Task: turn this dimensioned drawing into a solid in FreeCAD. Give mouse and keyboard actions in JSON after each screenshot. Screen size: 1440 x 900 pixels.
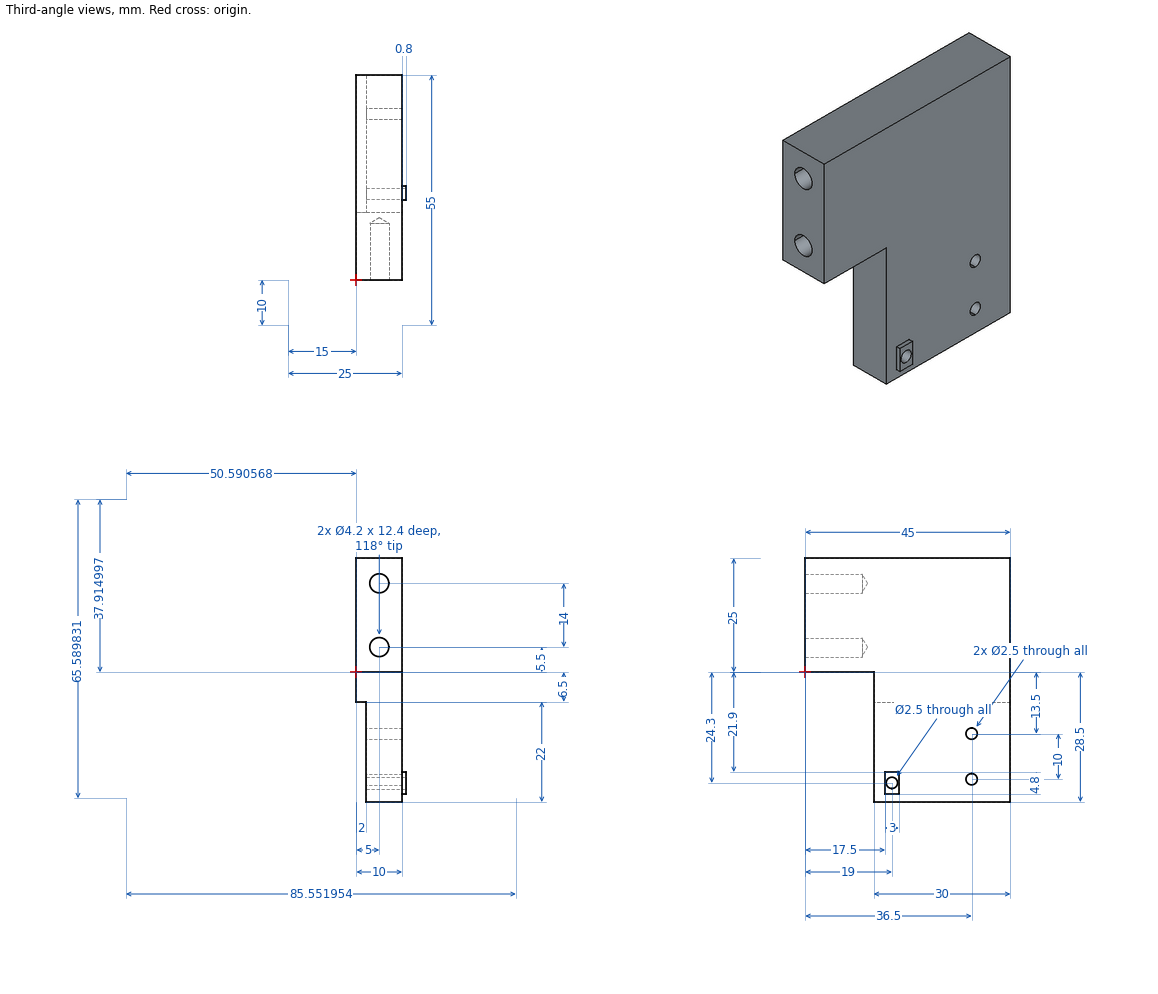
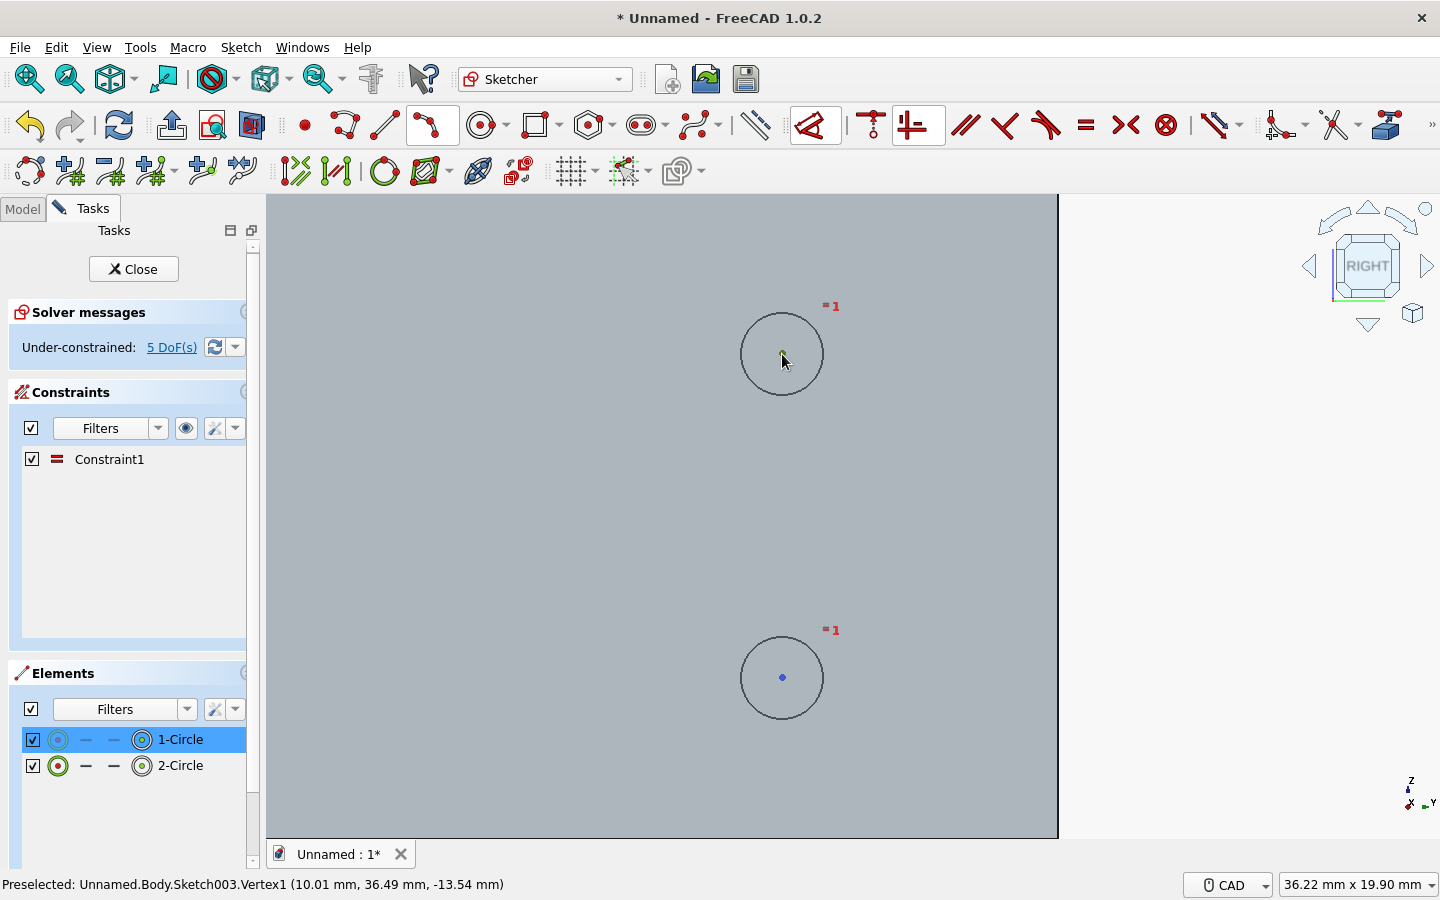
{"action": "left_click", "coordinate": [782, 678]}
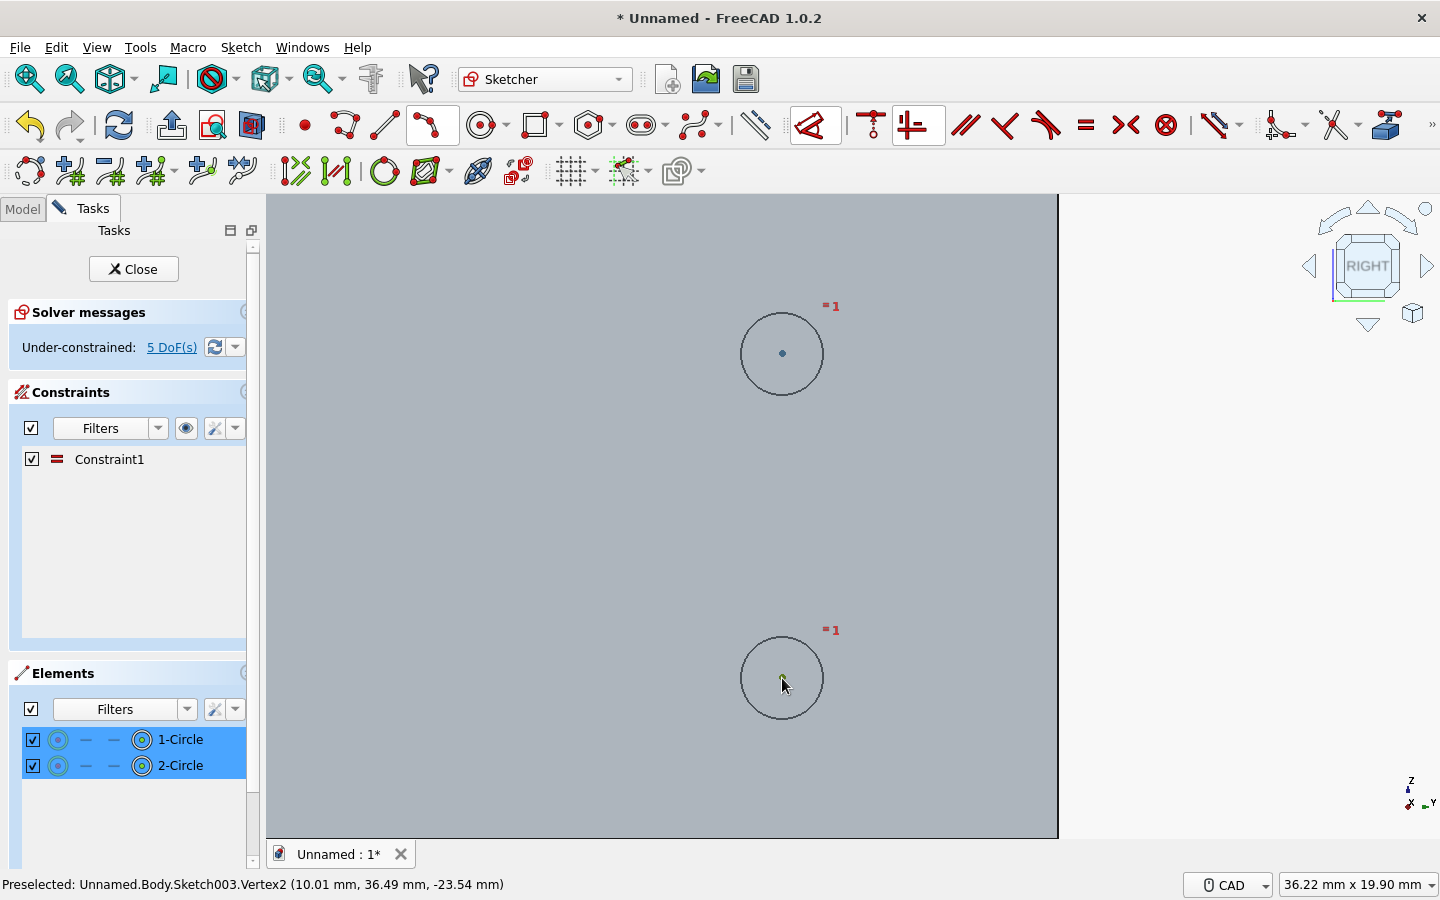
{"action": "key", "text": "v"}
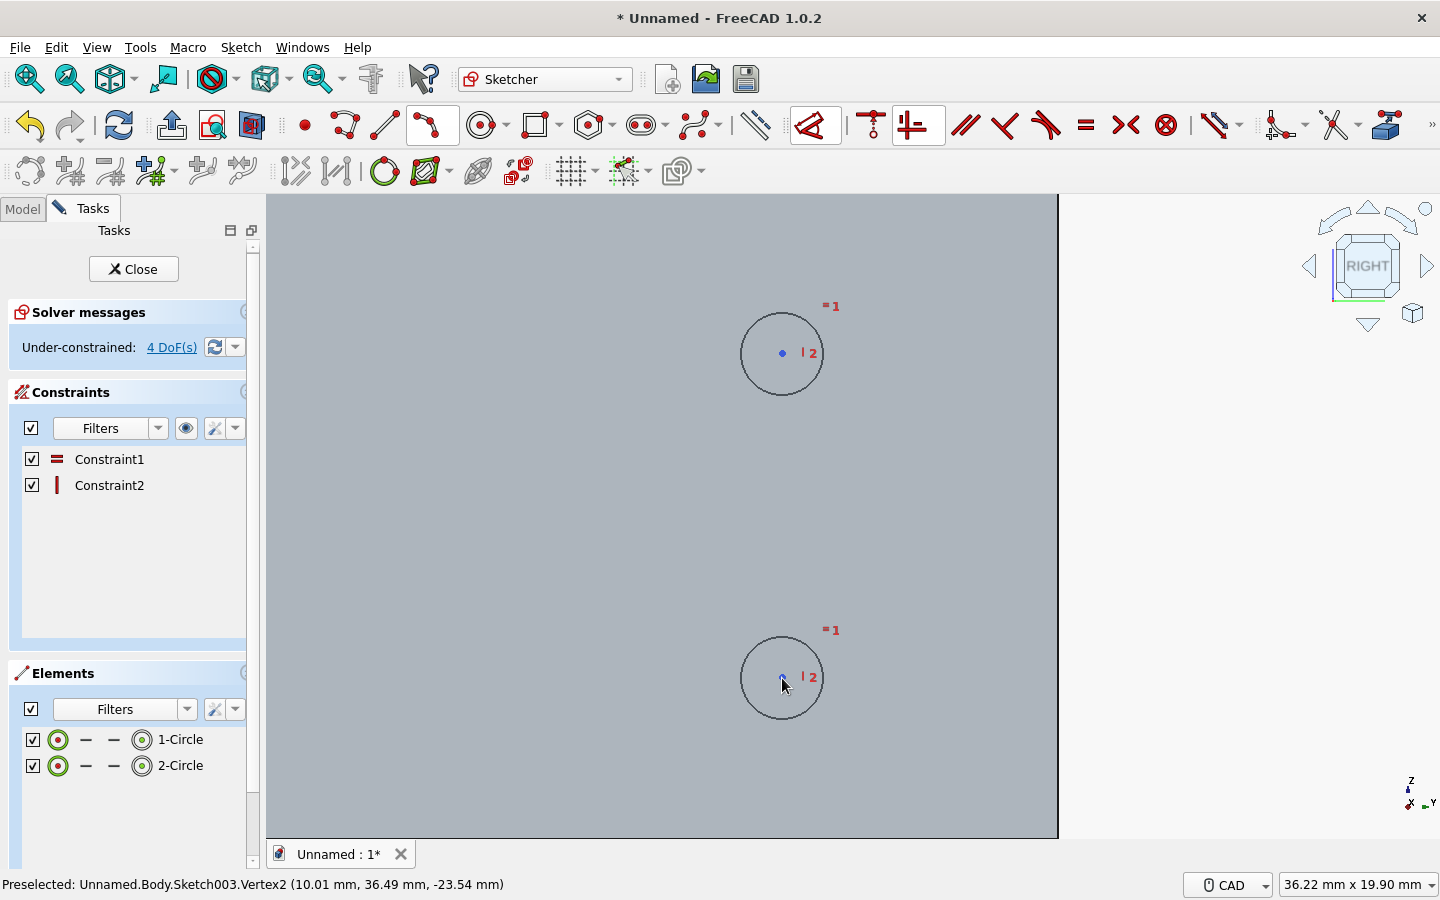
{"action": "left_click", "coordinate": [811, 325]}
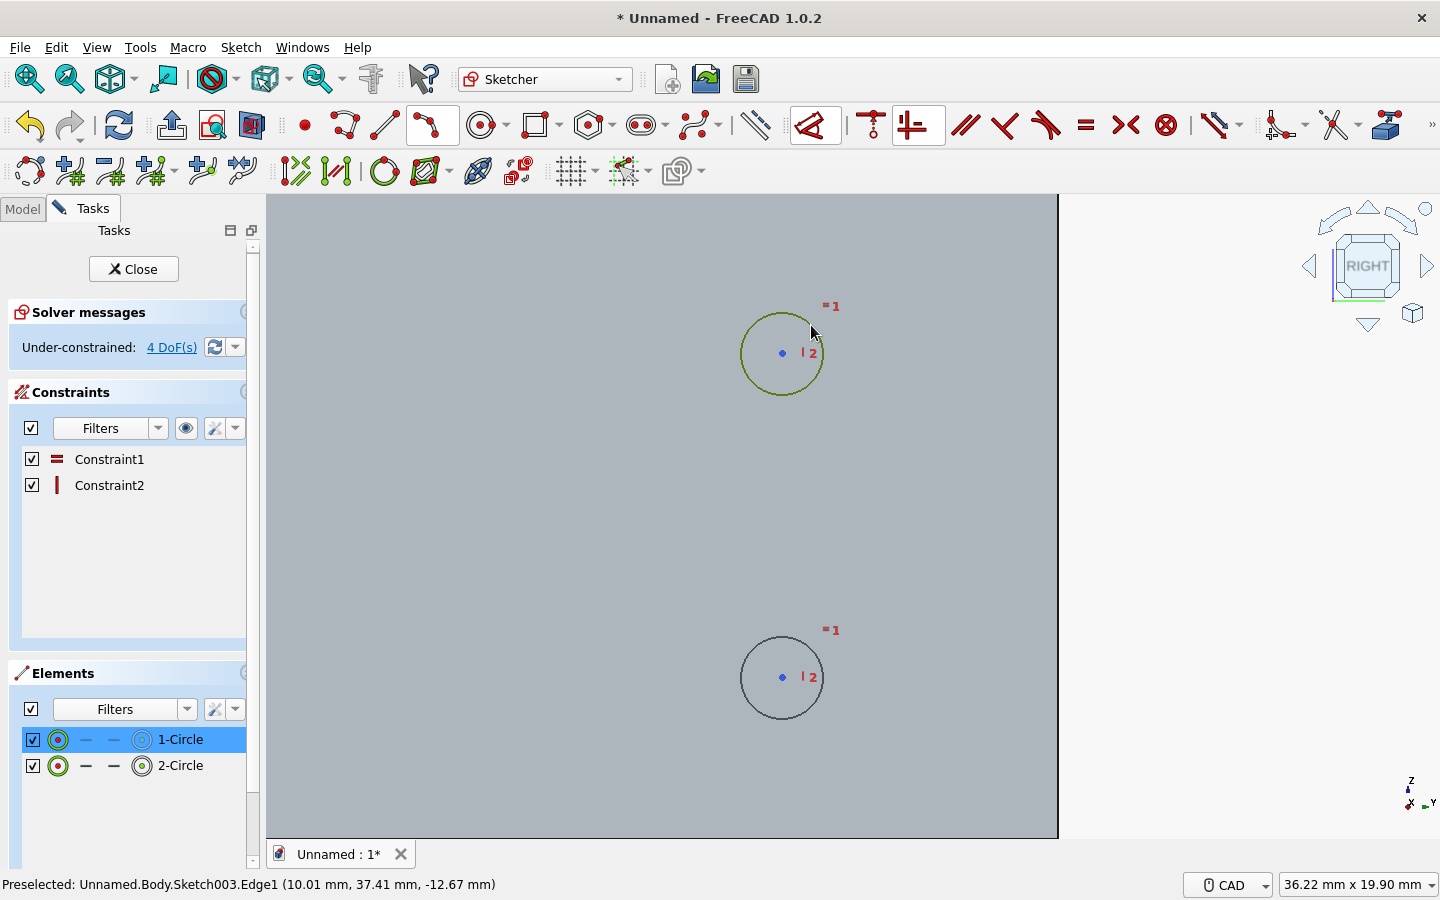
{"action": "left_click", "coordinate": [836, 126]}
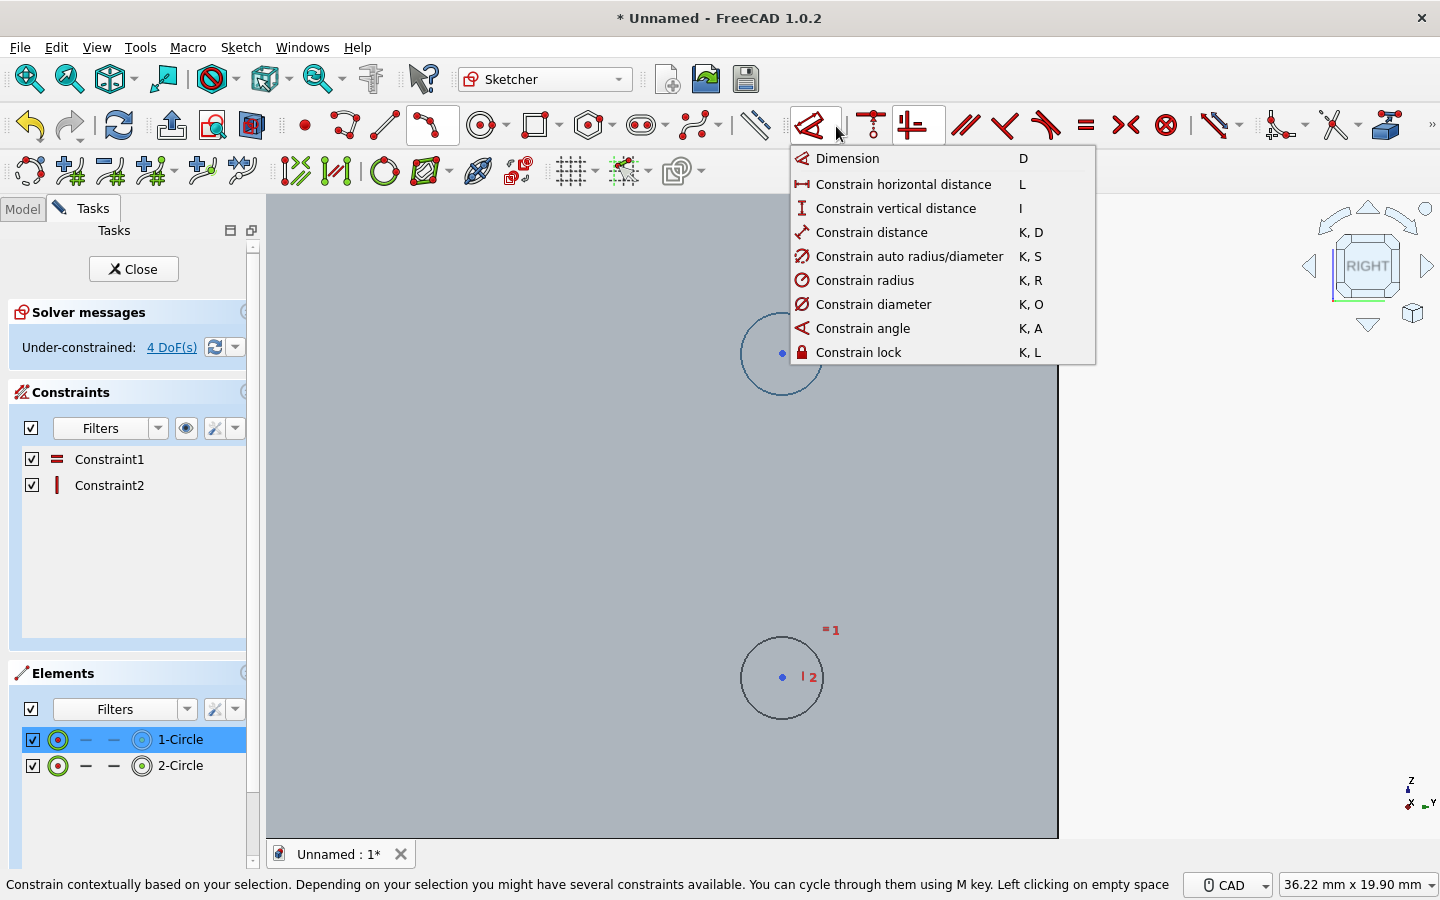
{"action": "left_click", "coordinate": [943, 304]}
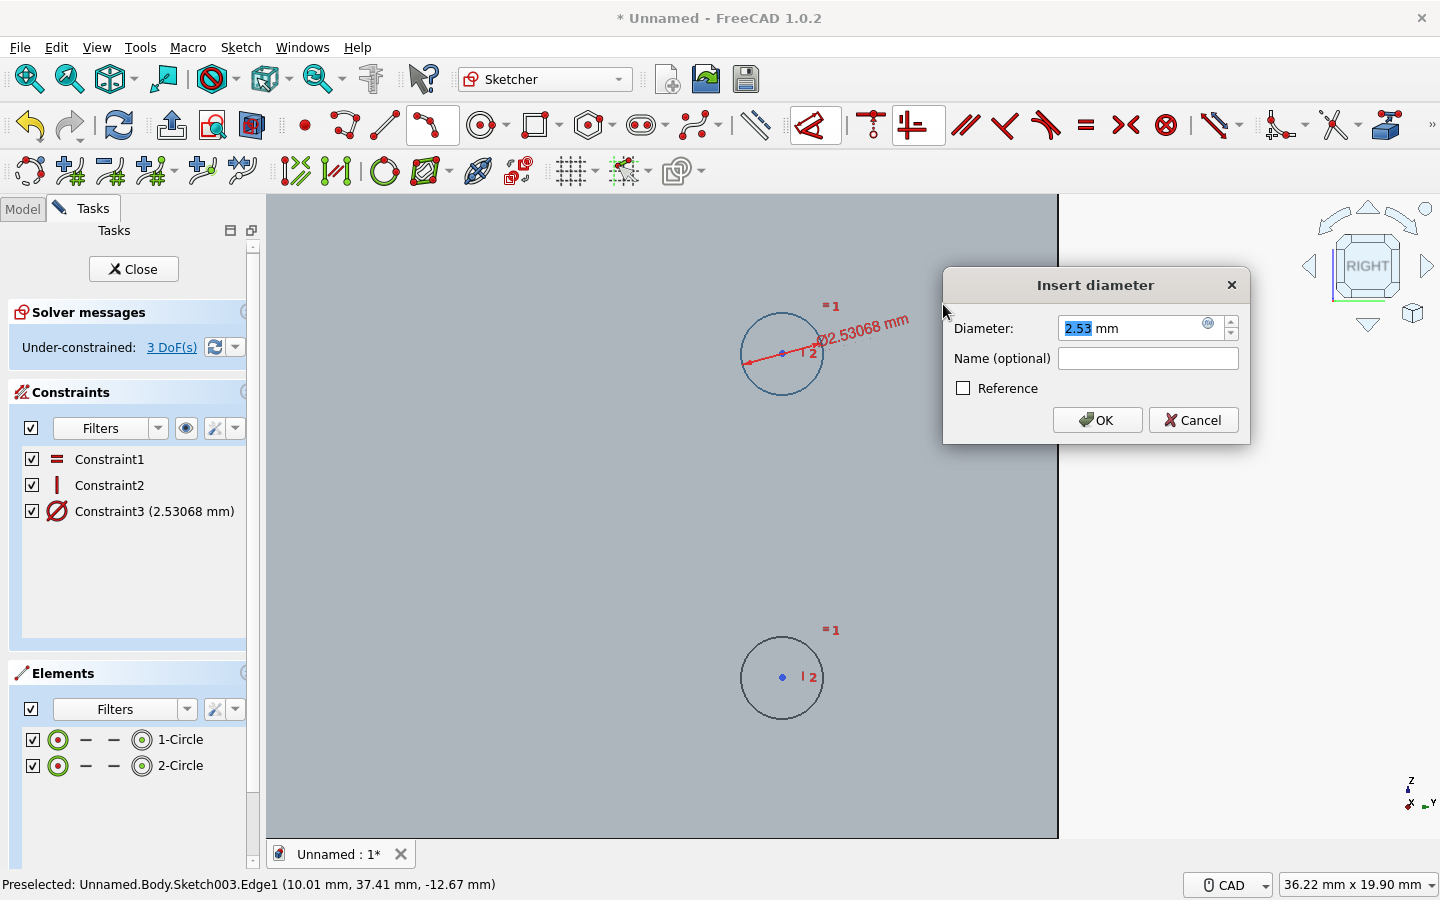
{"action": "type", "text": "2.5"}
{"action": "key", "text": "Return"}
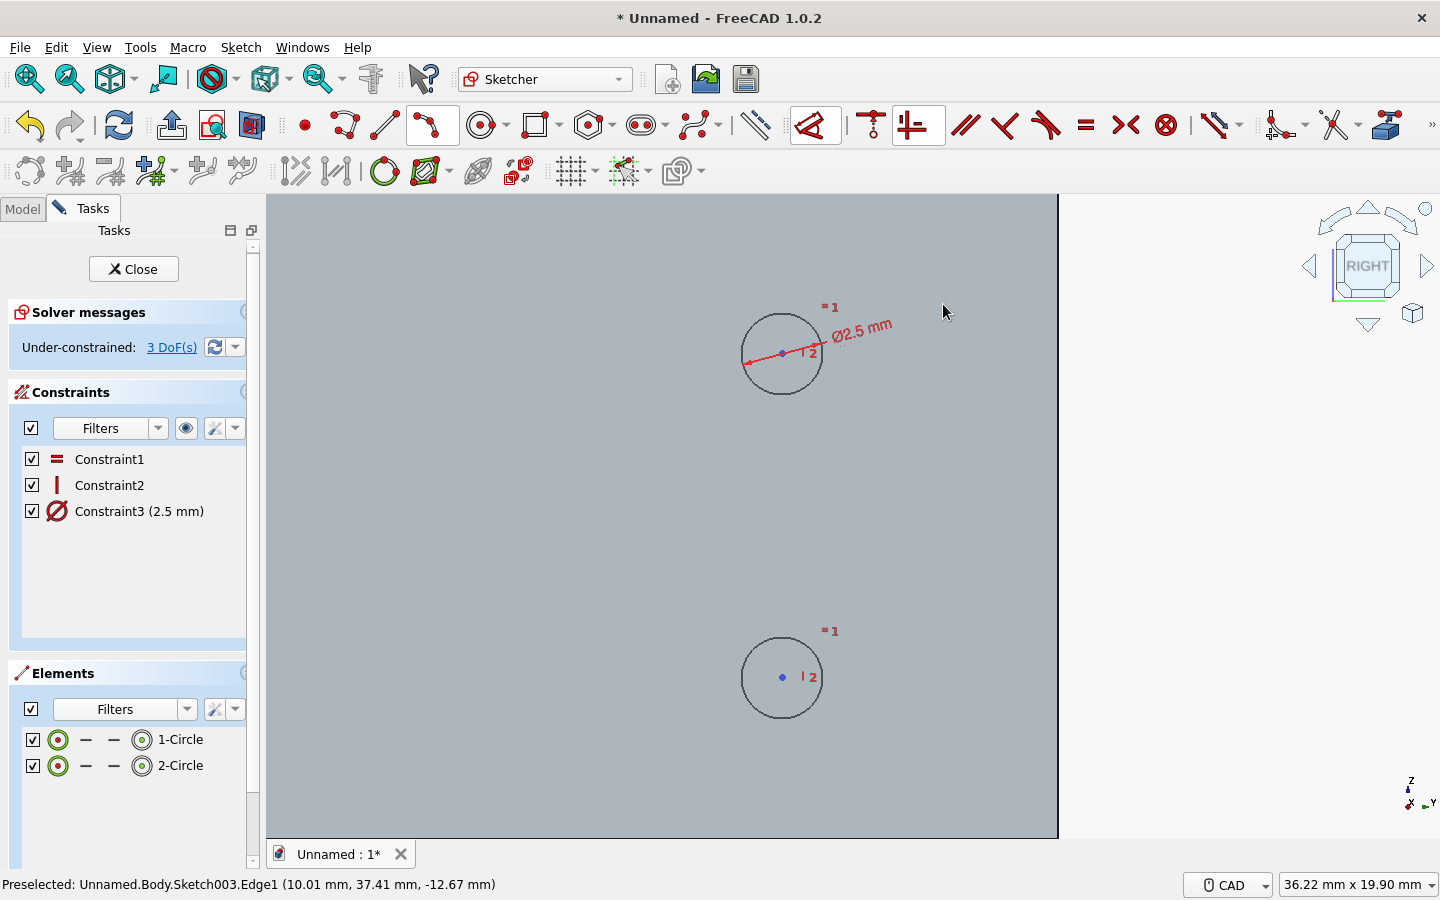
{"action": "left_click", "coordinate": [782, 354]}